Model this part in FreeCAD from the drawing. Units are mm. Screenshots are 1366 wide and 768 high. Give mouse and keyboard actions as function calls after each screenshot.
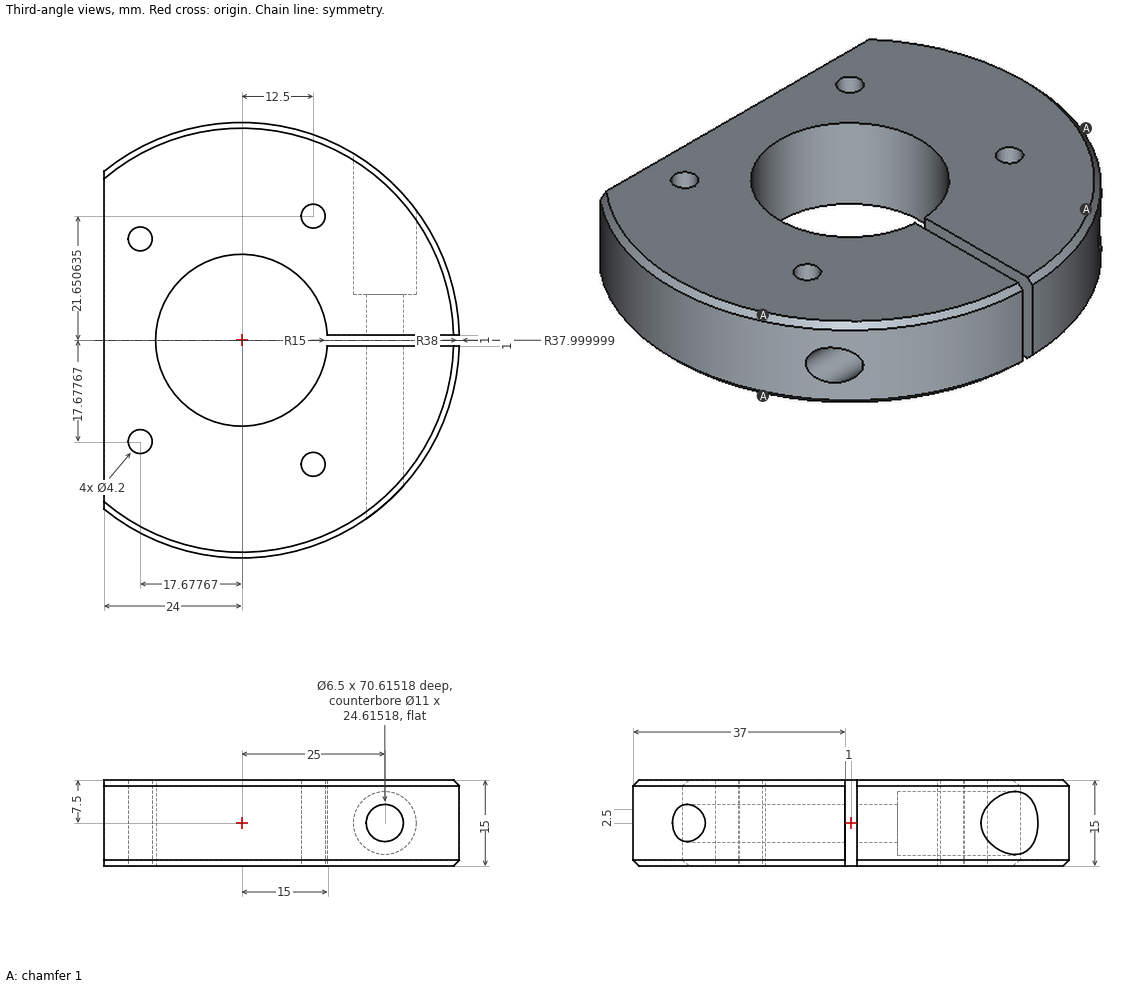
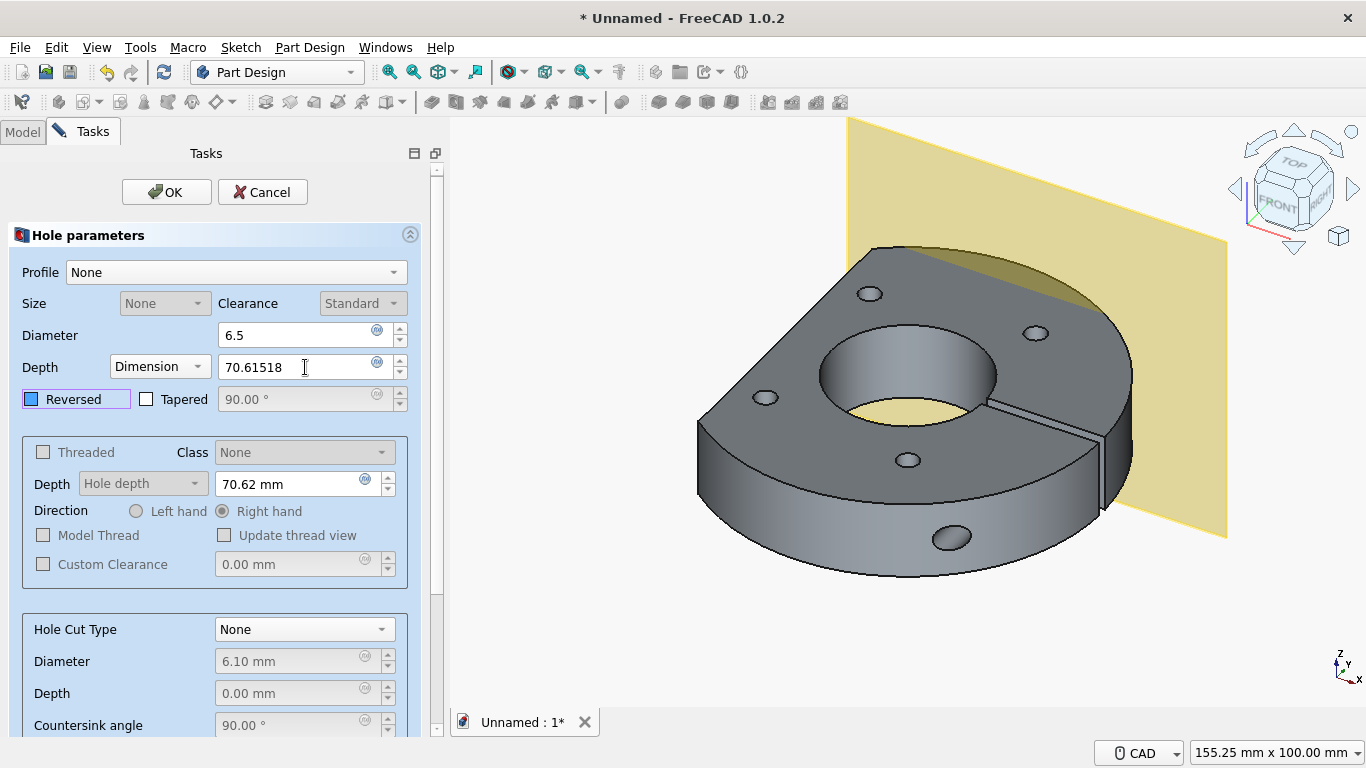
click(30, 399)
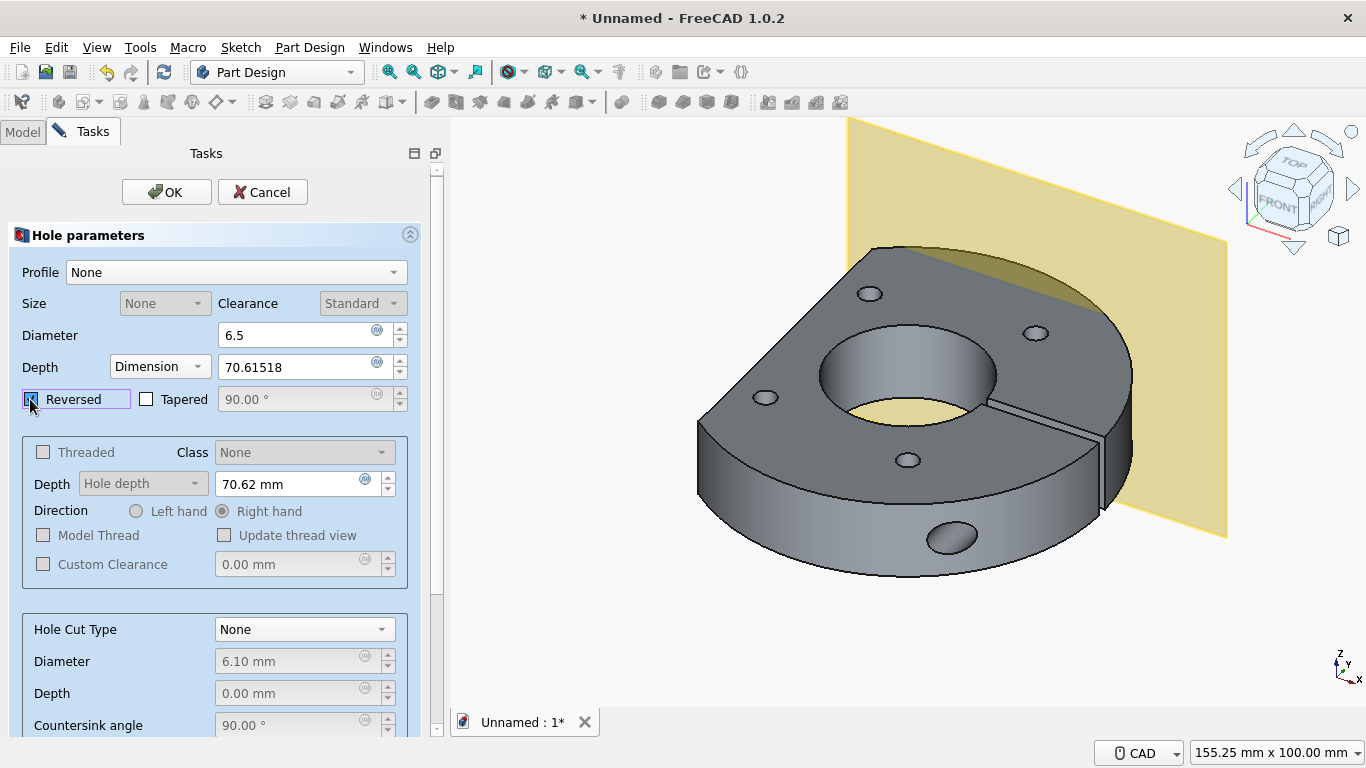
click(306, 630)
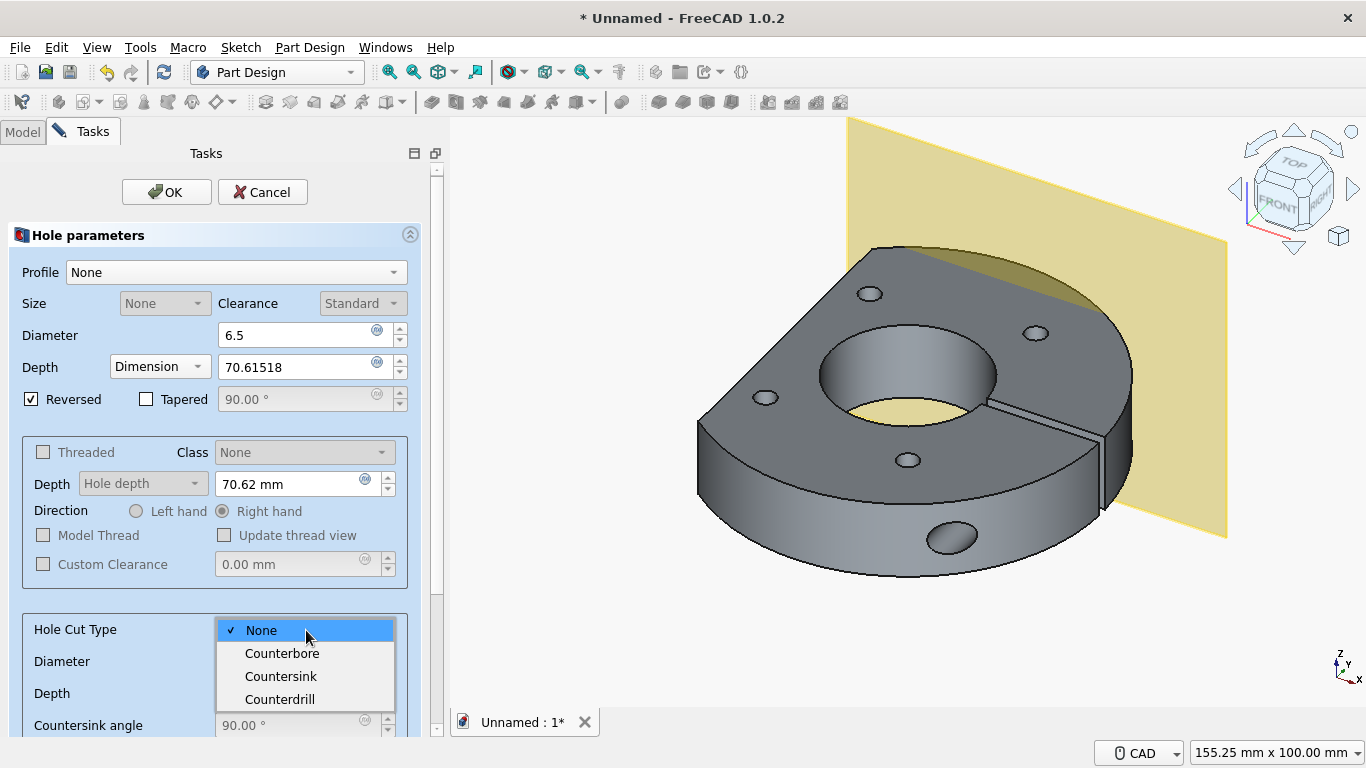
click(304, 654)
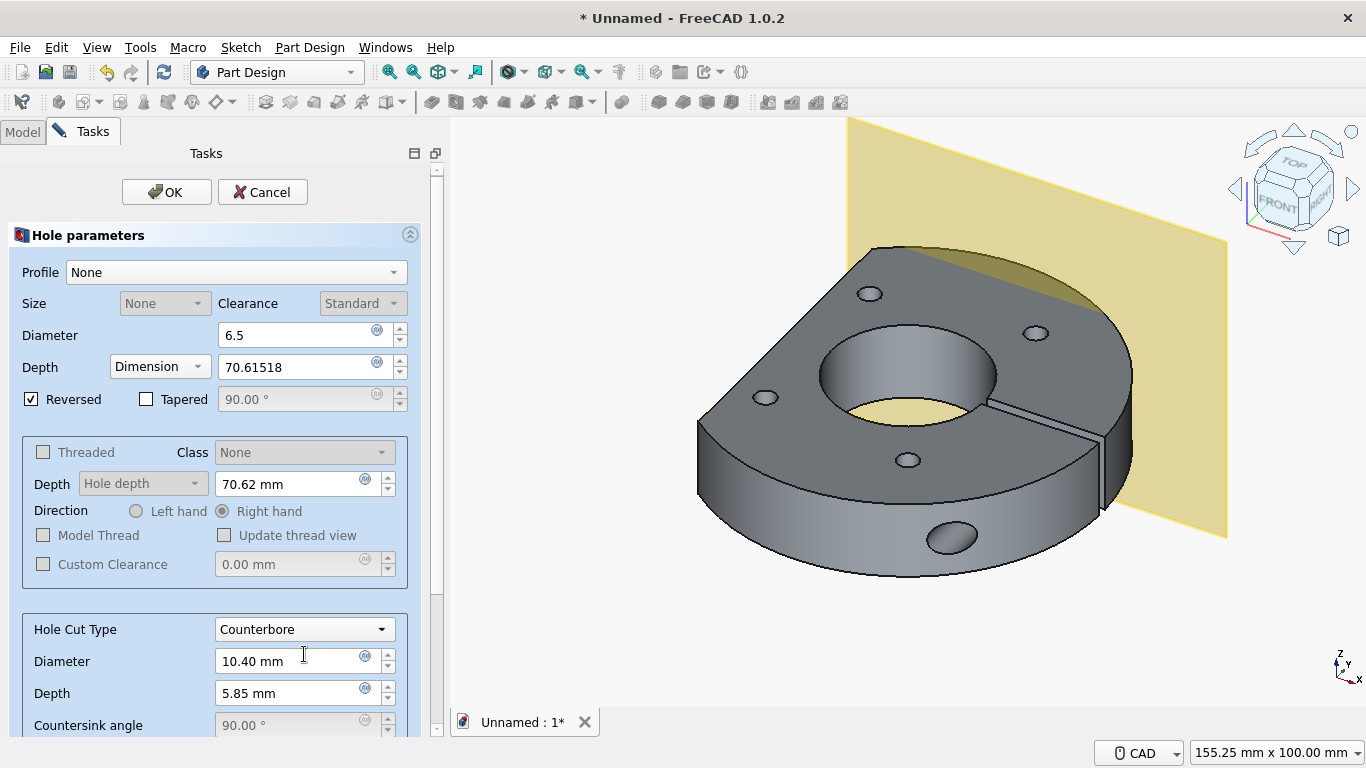
triple_click(298, 661)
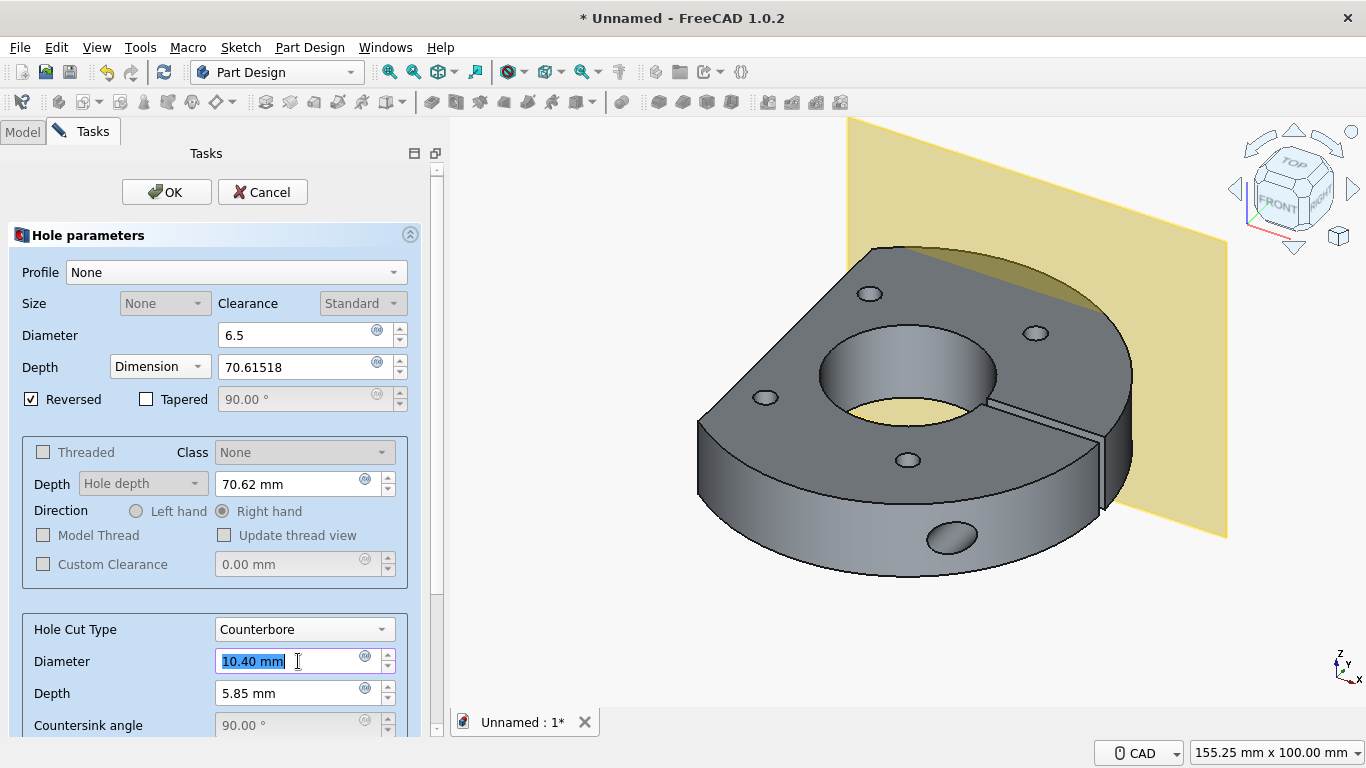
text(11)
key(Tab)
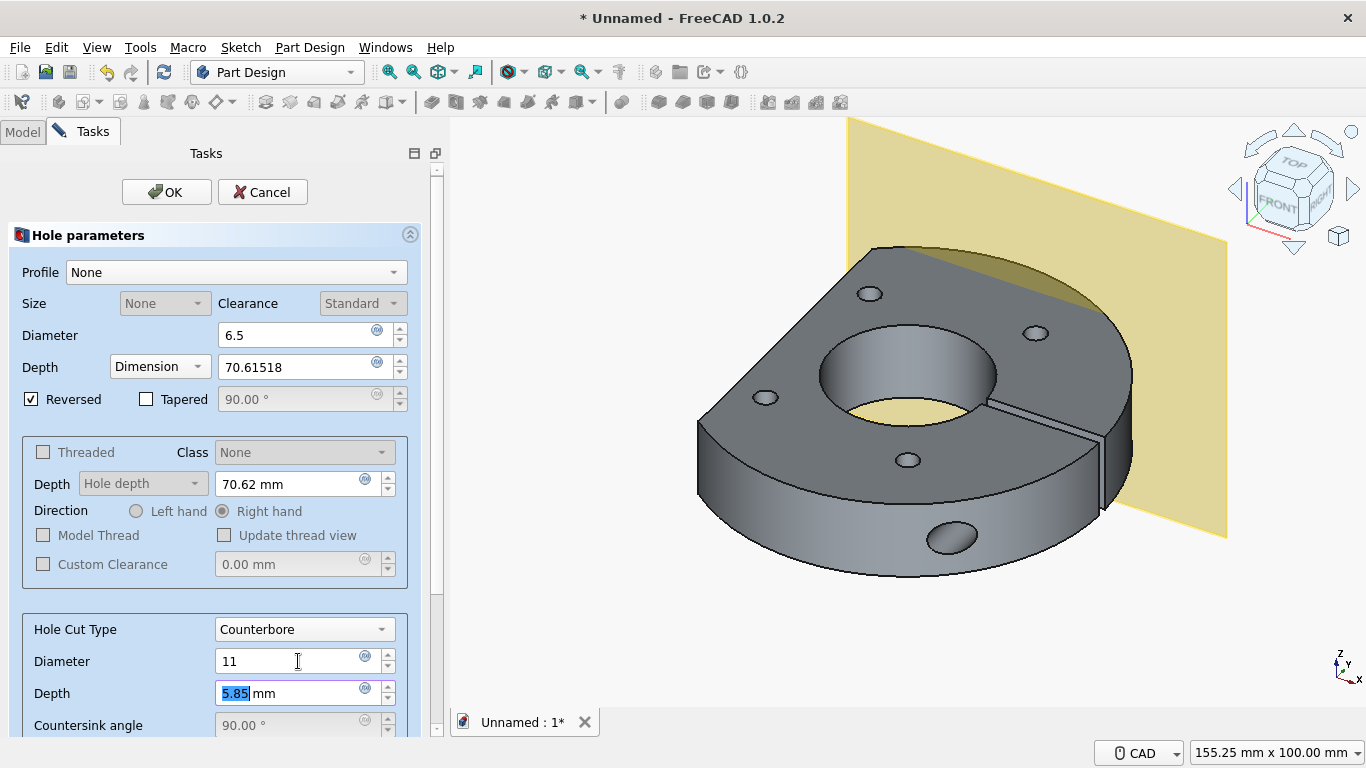
text(24.61518)
key(Tab)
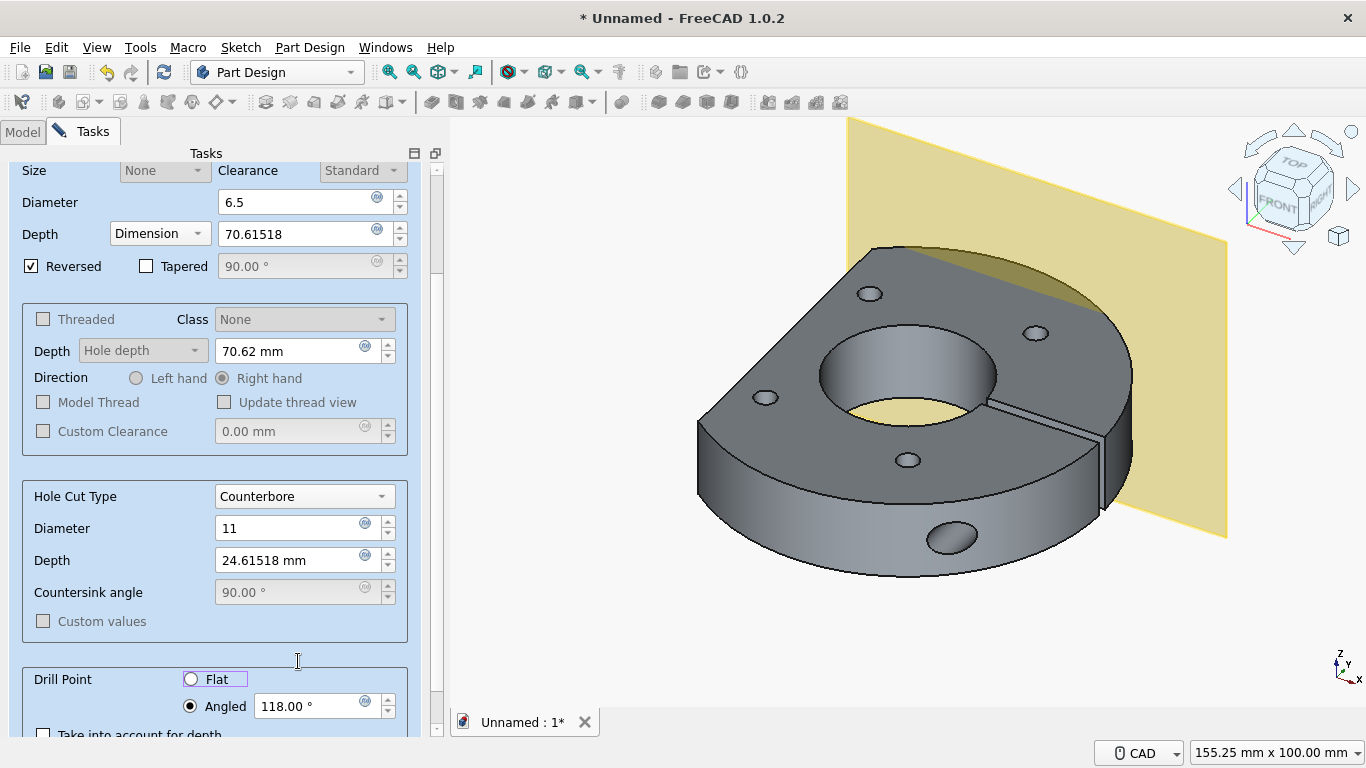
click(191, 679)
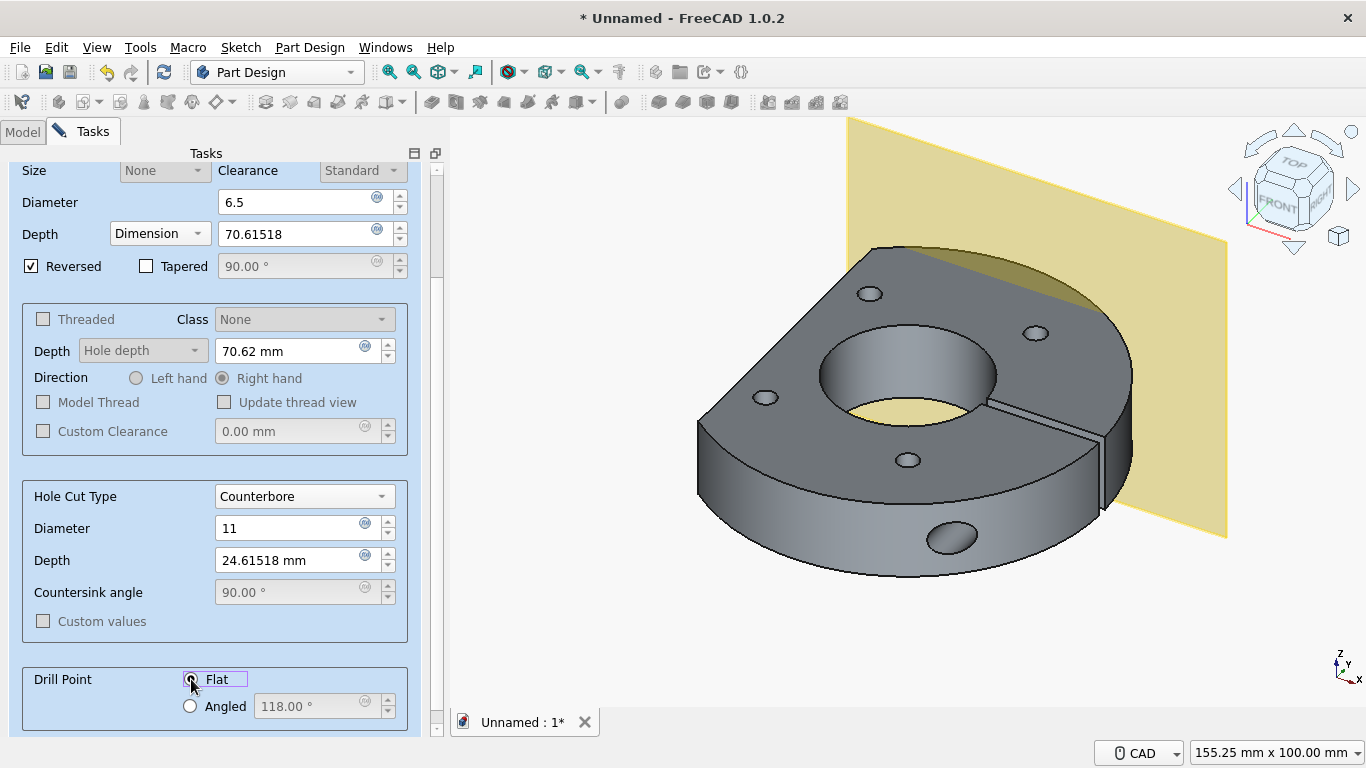
scroll(437, 450, up, 3)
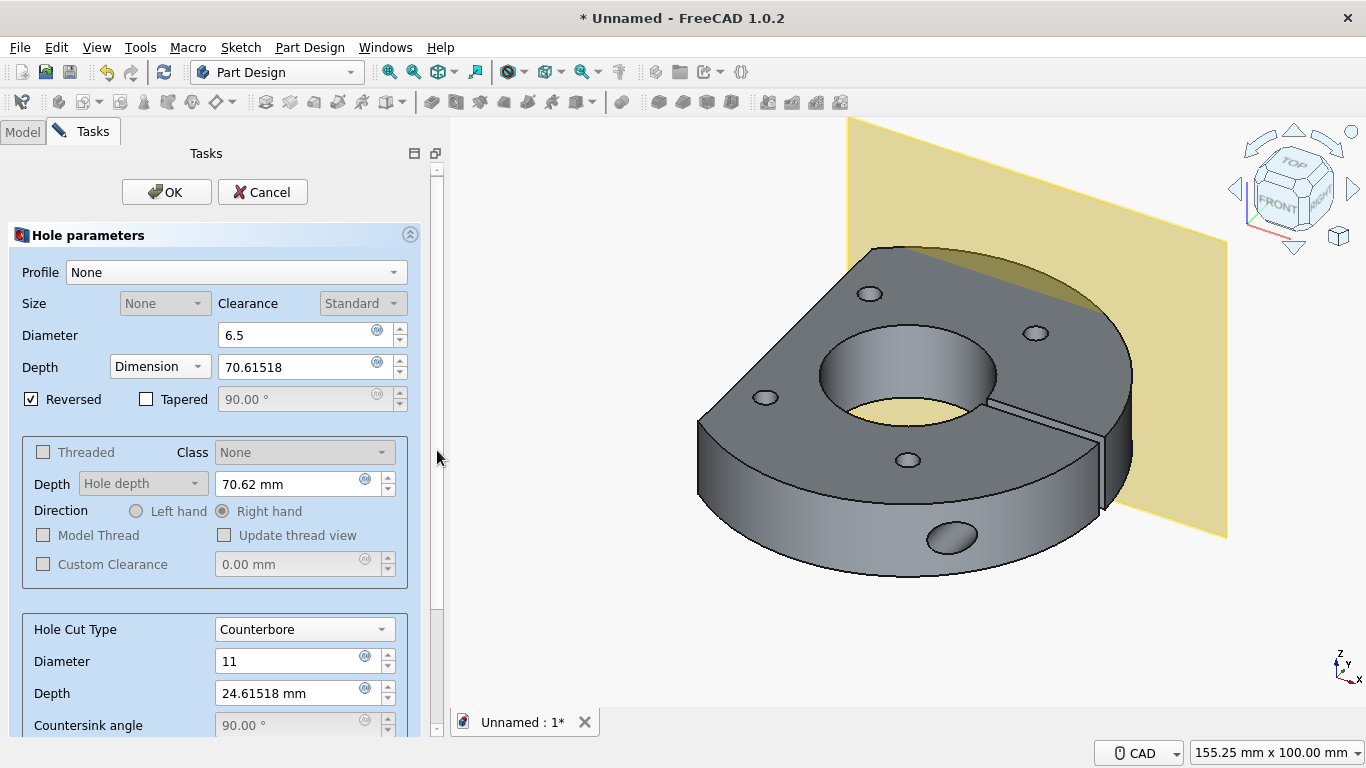
click(167, 192)